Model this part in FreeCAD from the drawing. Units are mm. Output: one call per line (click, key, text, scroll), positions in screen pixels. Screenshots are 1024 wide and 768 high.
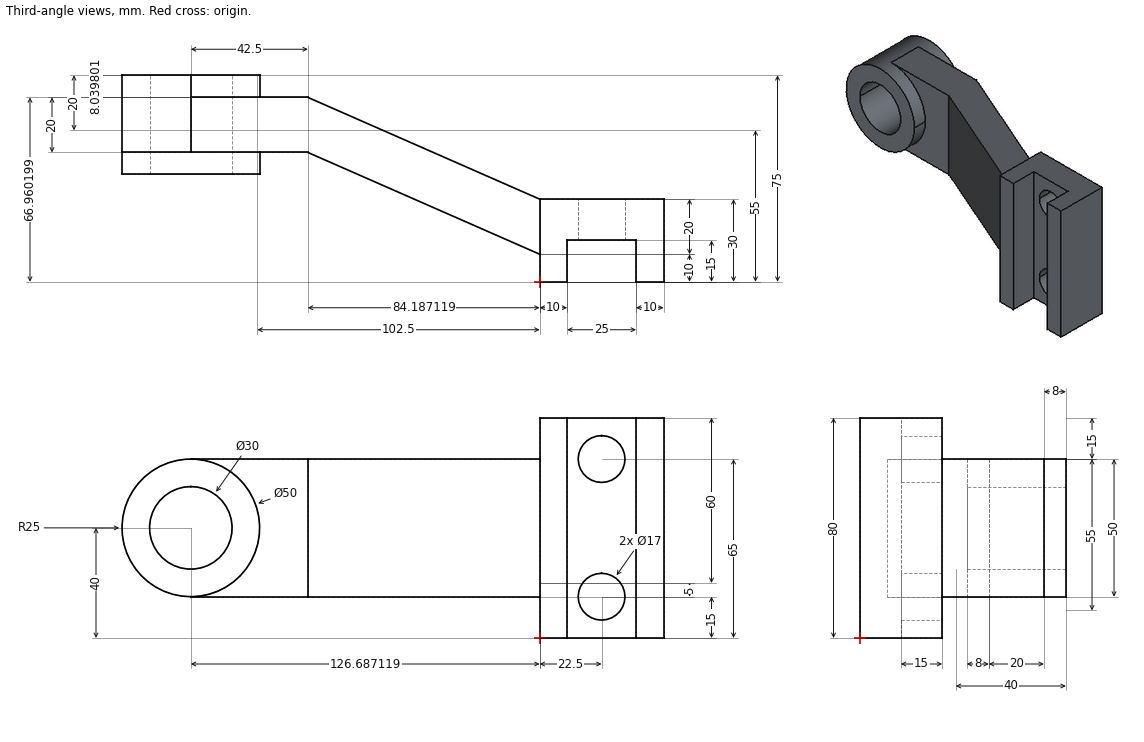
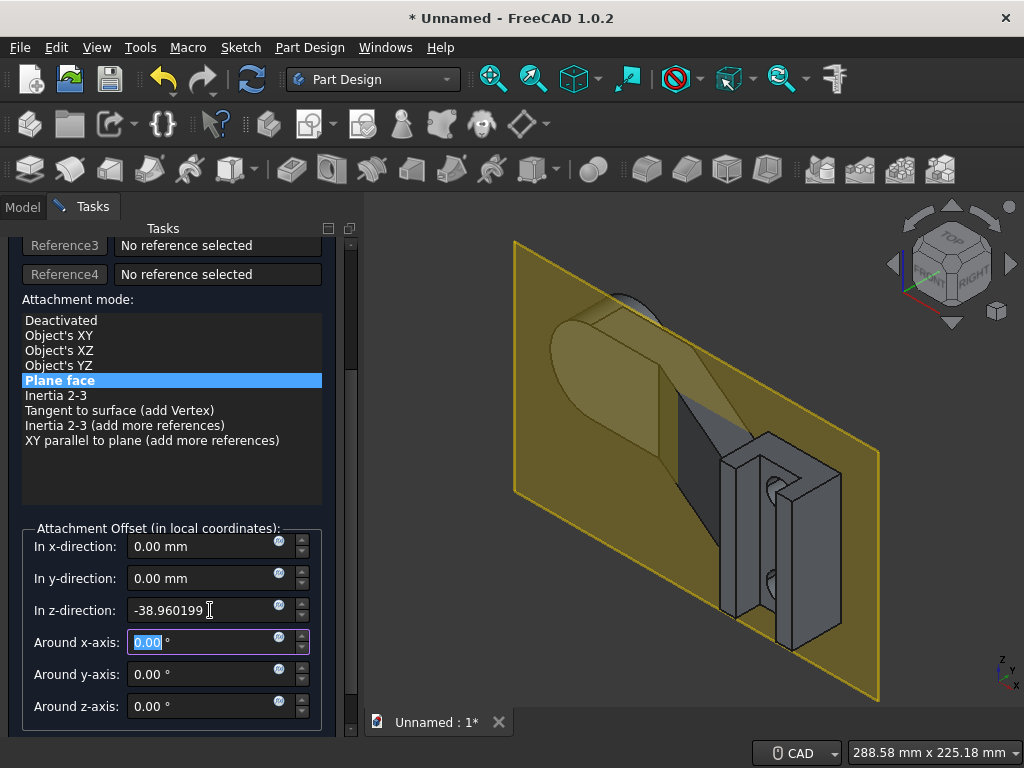
scroll(351, 487, up, 4)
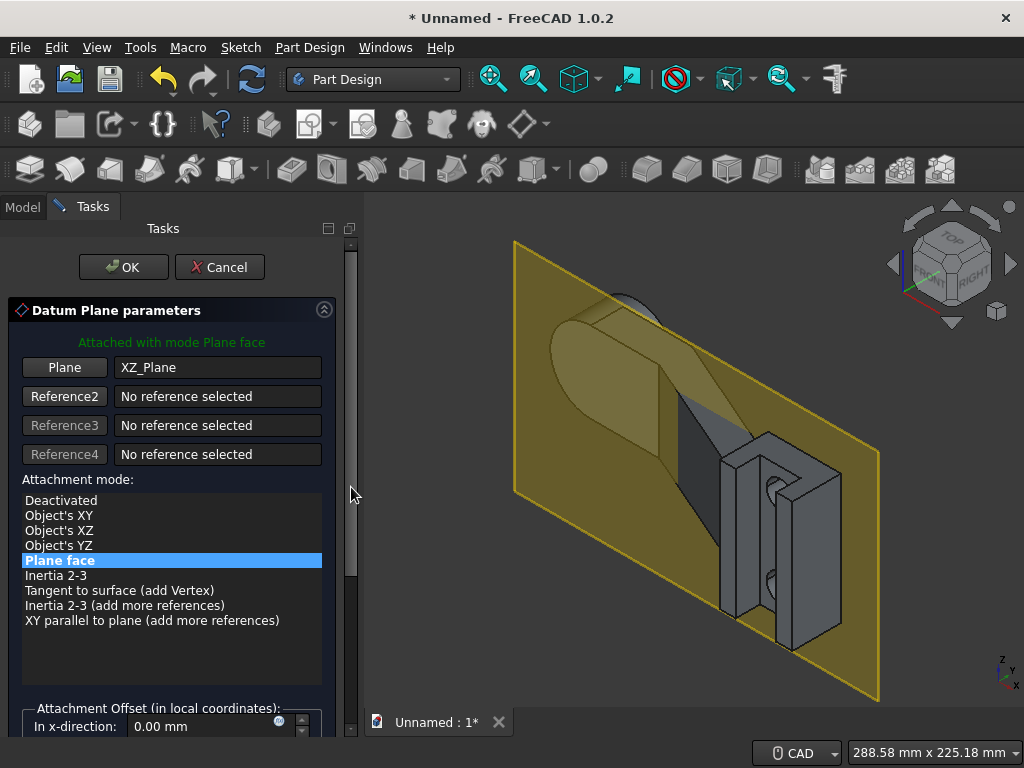
click(124, 267)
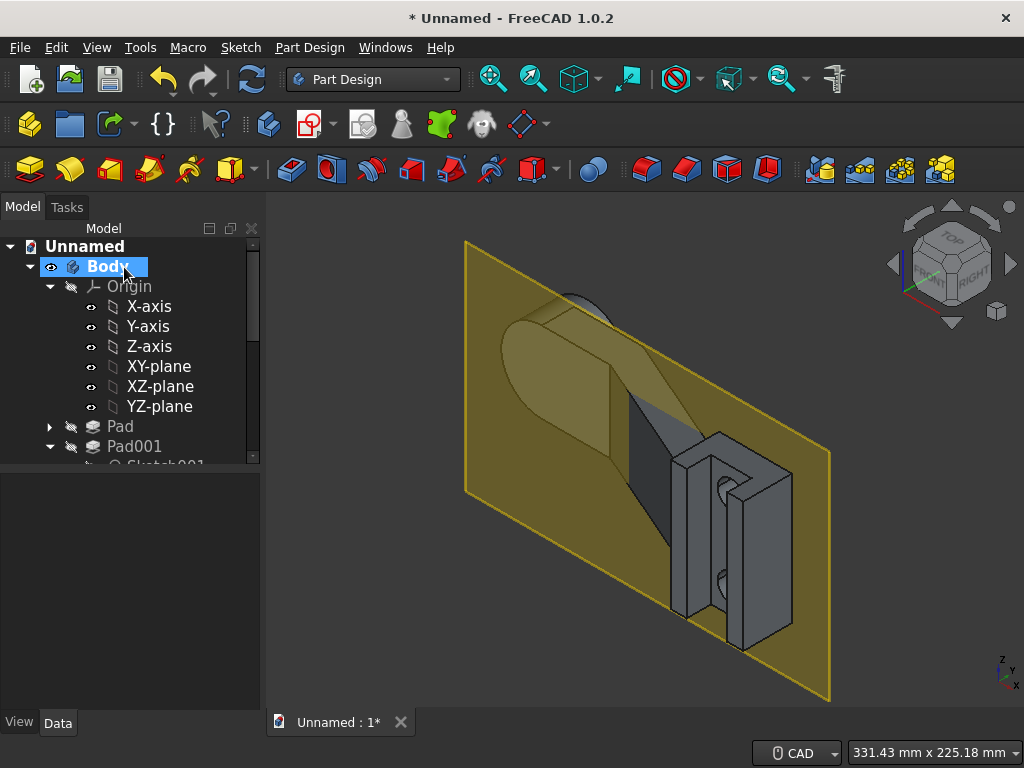
scroll(100, 342, down, 3)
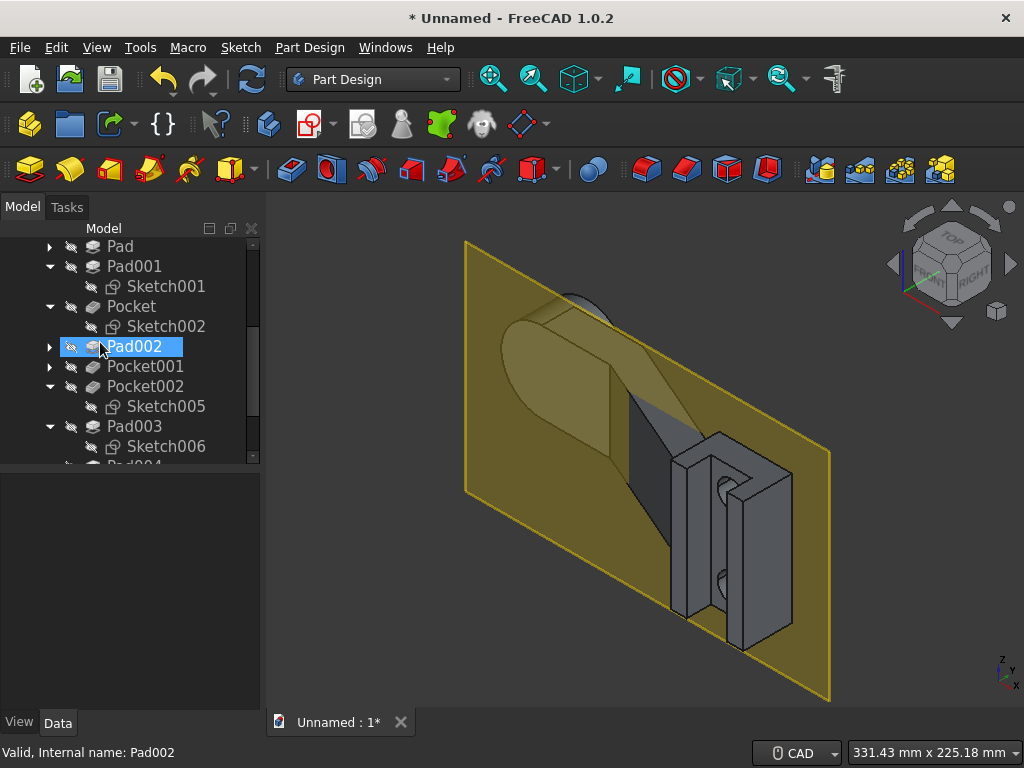
scroll(140, 342, up, 15)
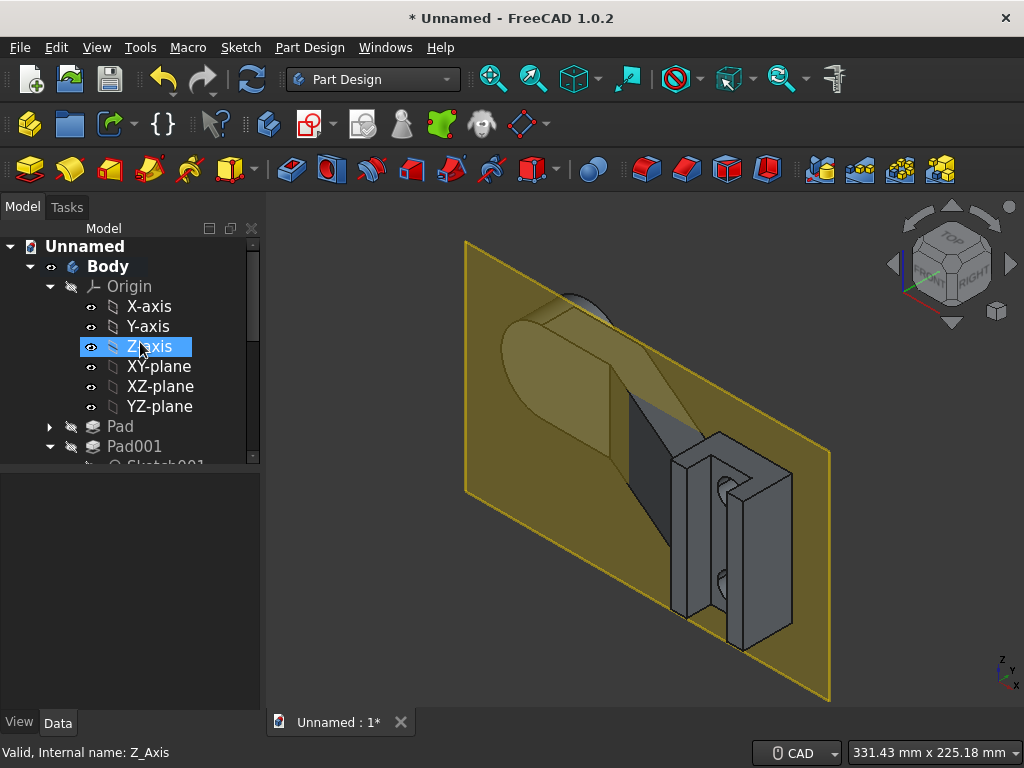
scroll(100, 342, down, 6)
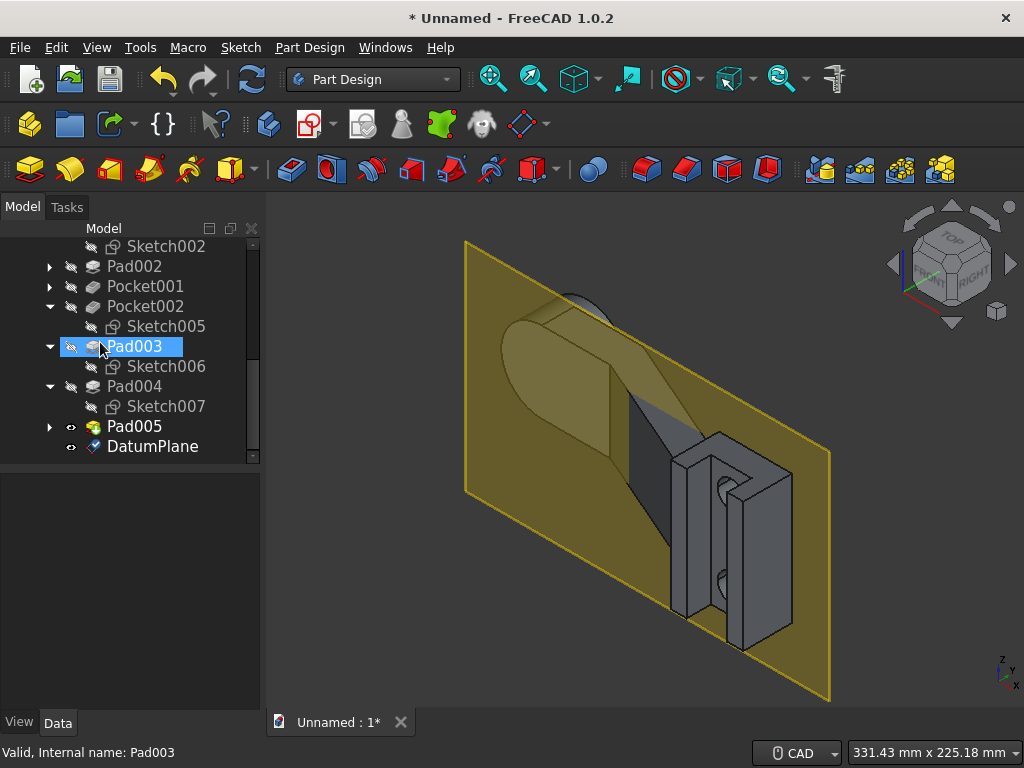
click(116, 447)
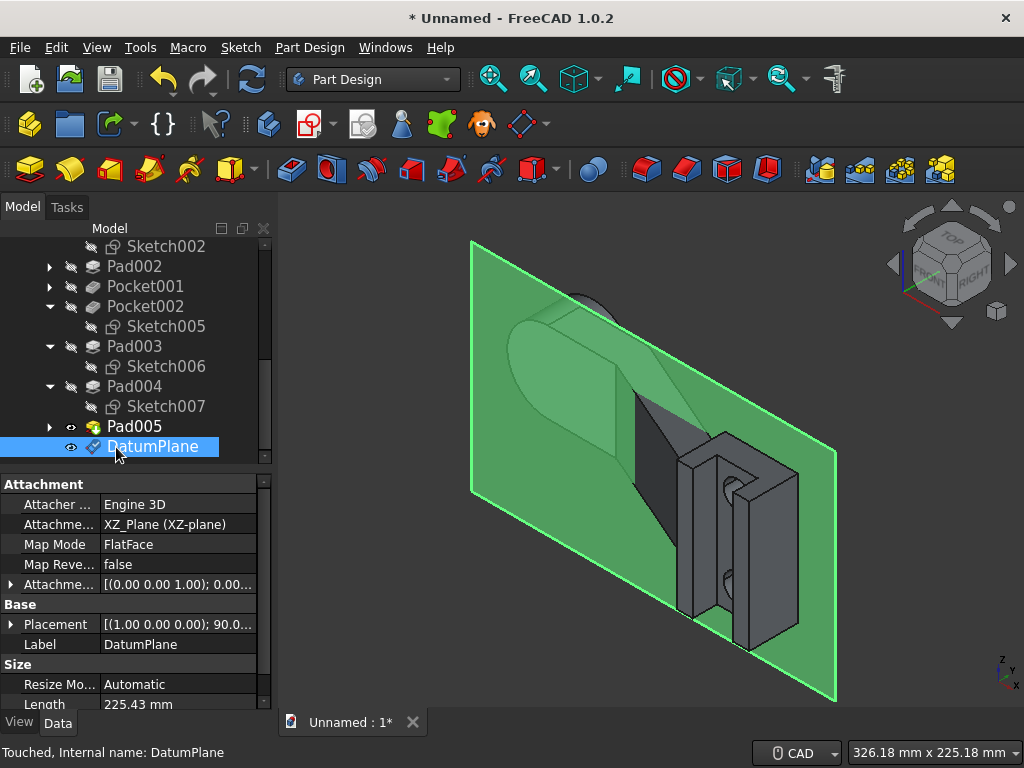
click(310, 124)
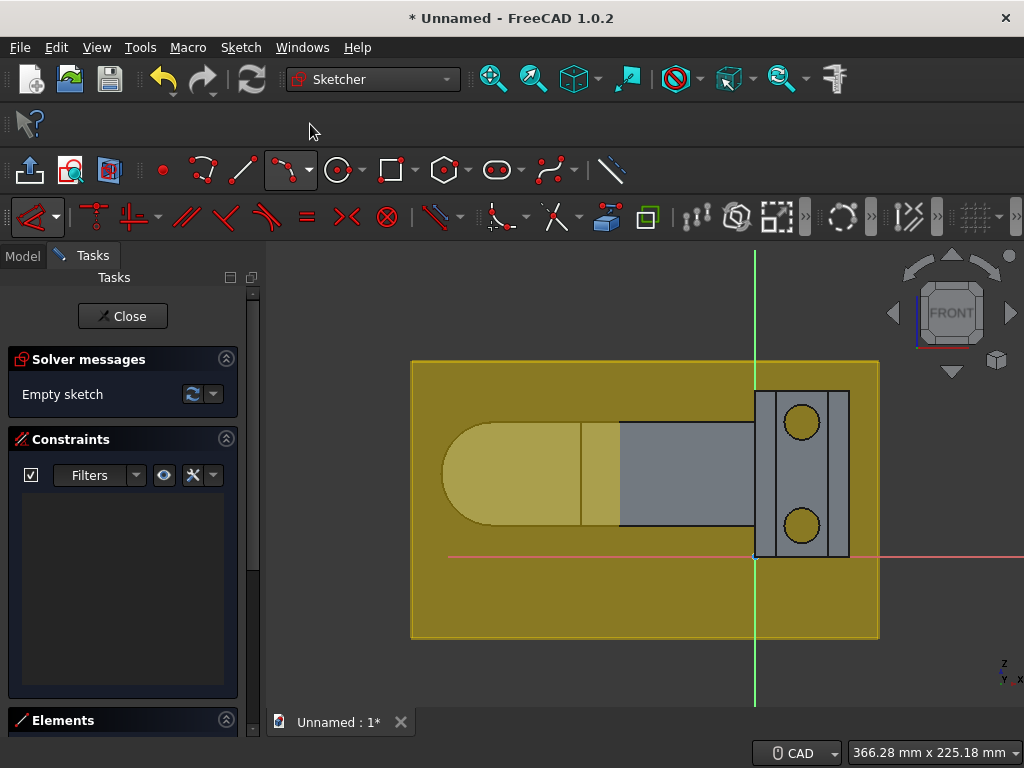
key(q)
key(s)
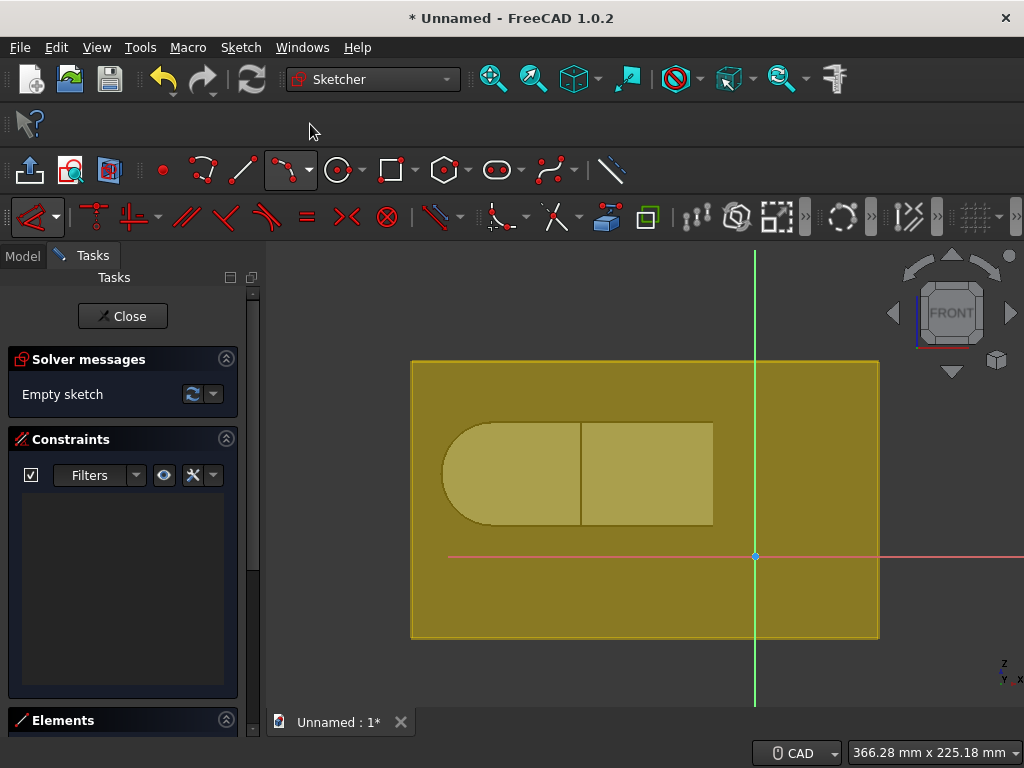
scroll(445, 474, up, 5)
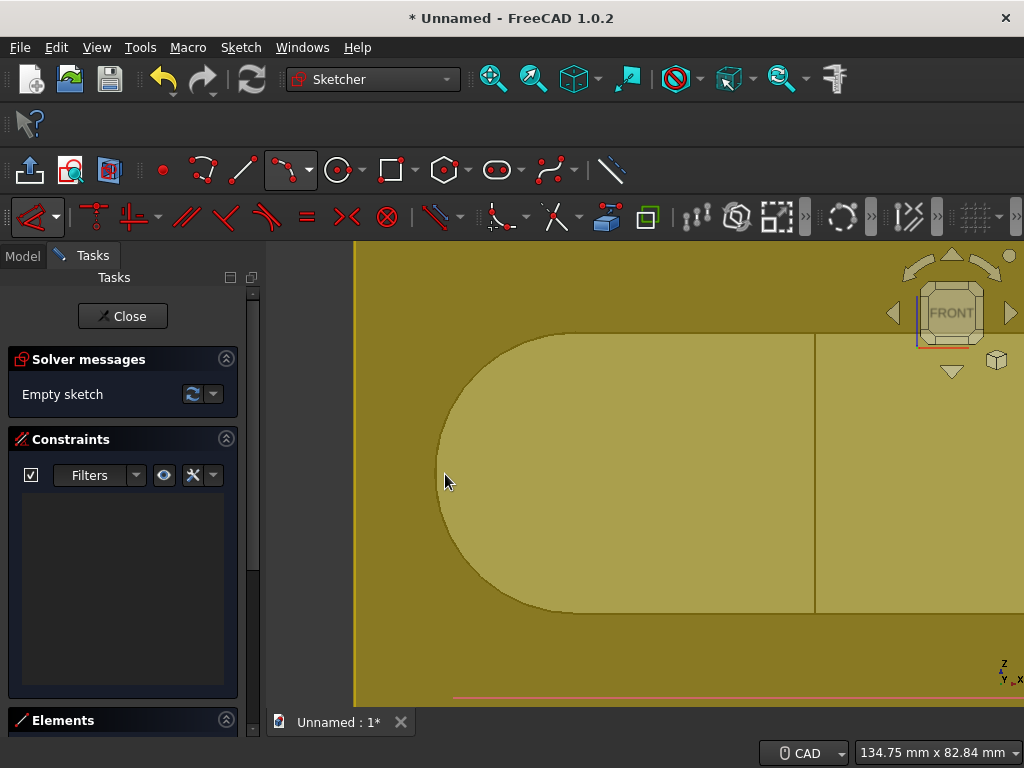
key(g)
key(c)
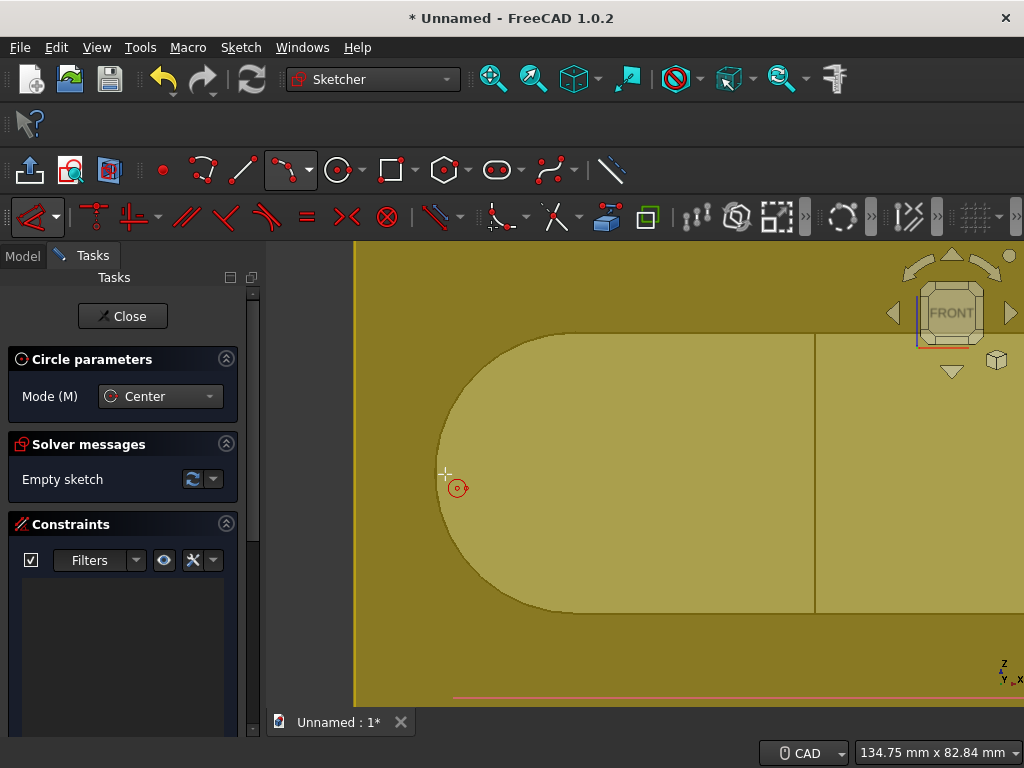
click(576, 473)
move(675, 374)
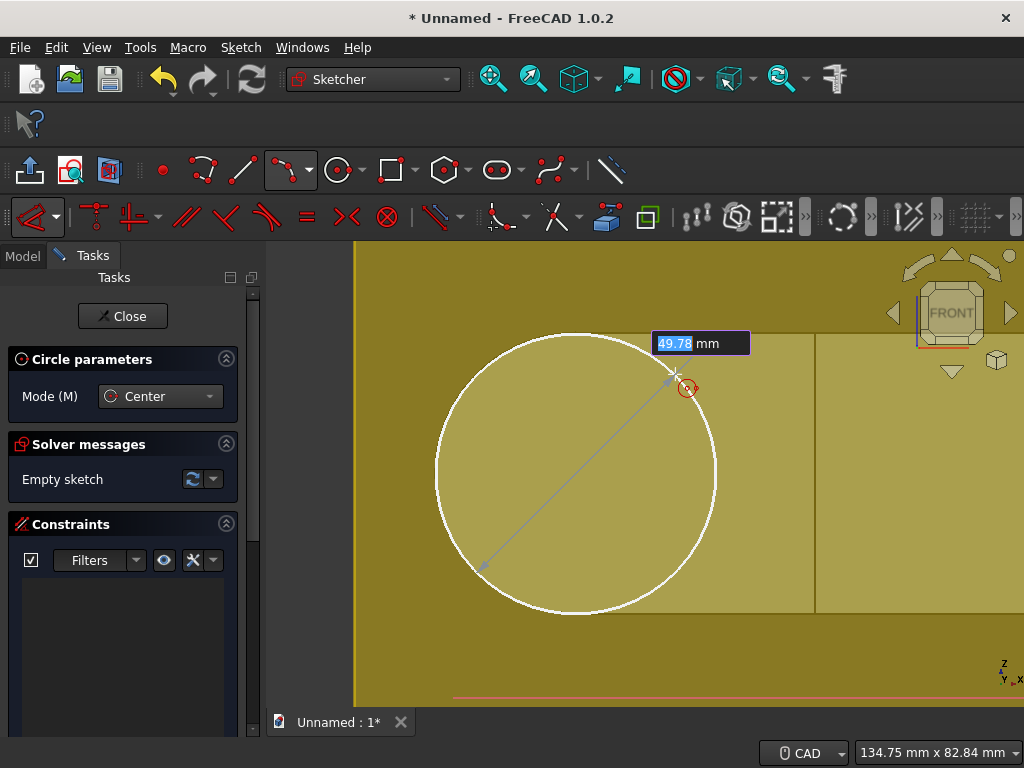
text(50)
key(Return)
key(Escape)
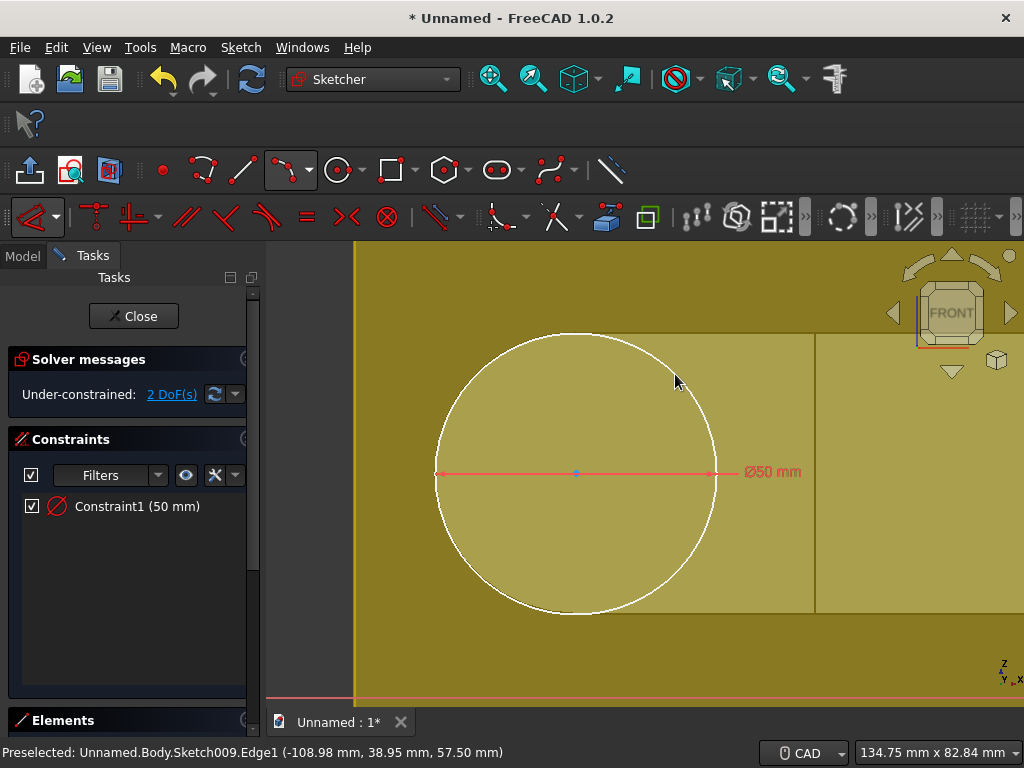
click(576, 474)